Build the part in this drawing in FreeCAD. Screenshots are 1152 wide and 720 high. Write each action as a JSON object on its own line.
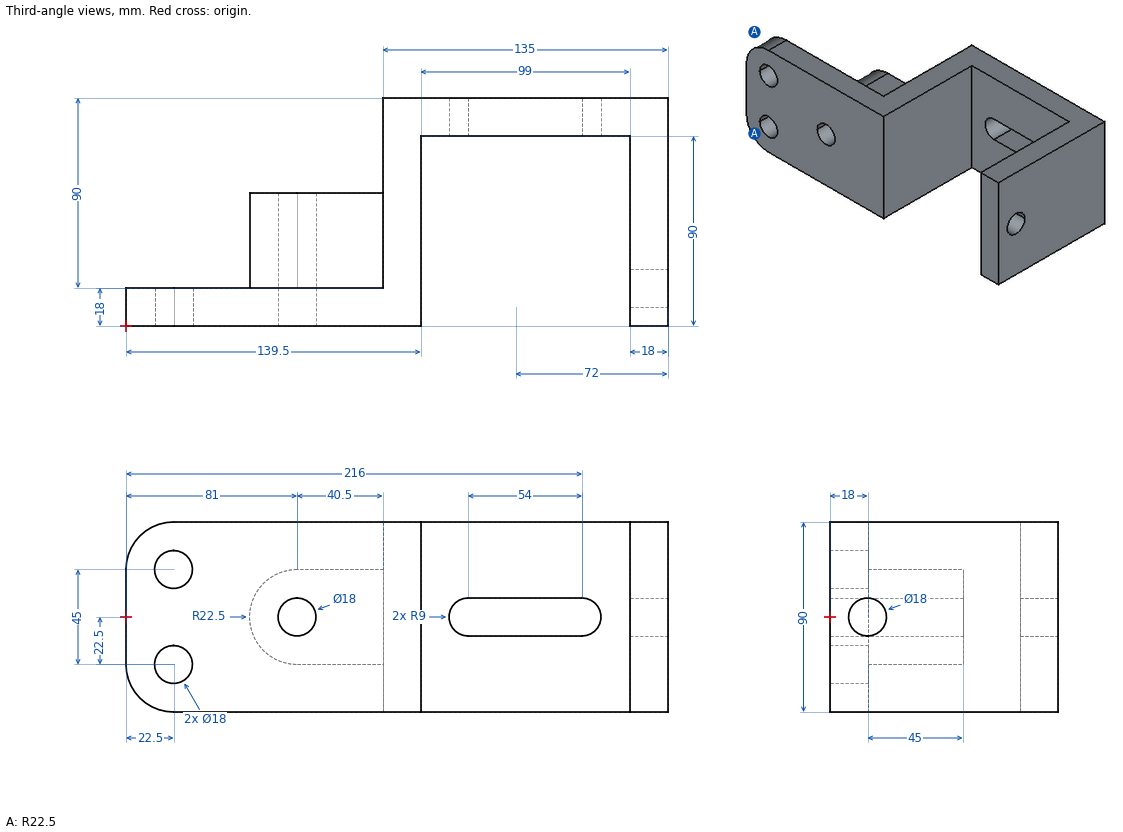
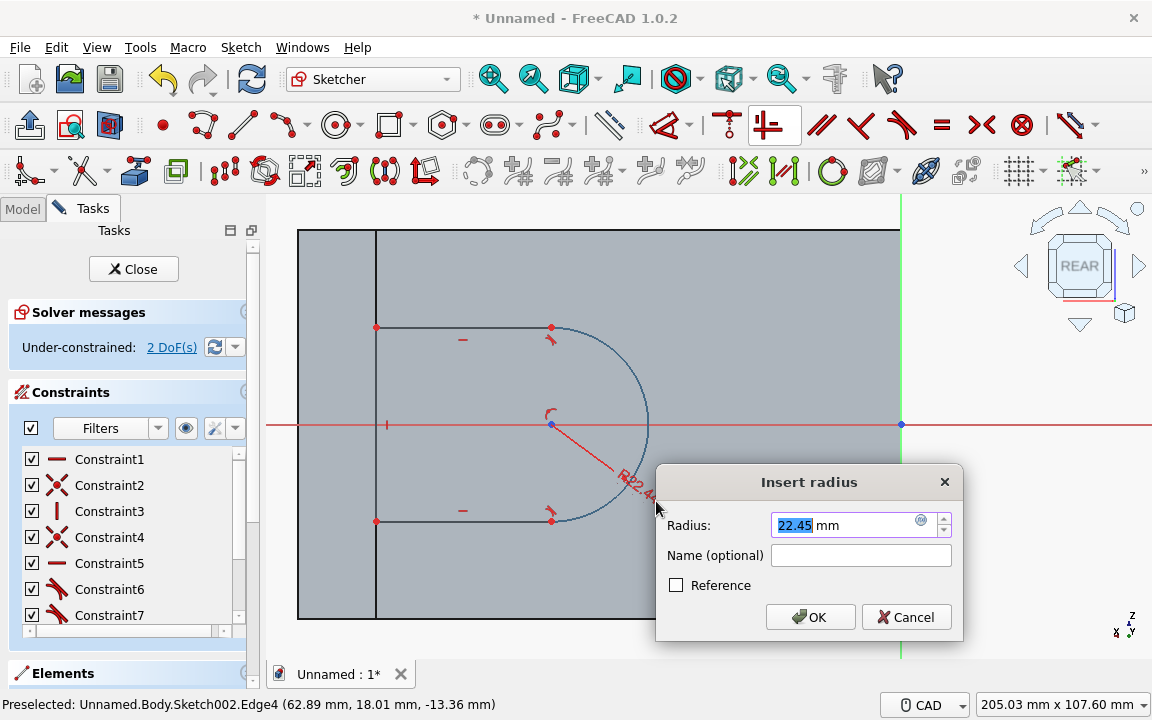
{"action": "type", "text": "22.5"}
{"action": "key", "text": "Return"}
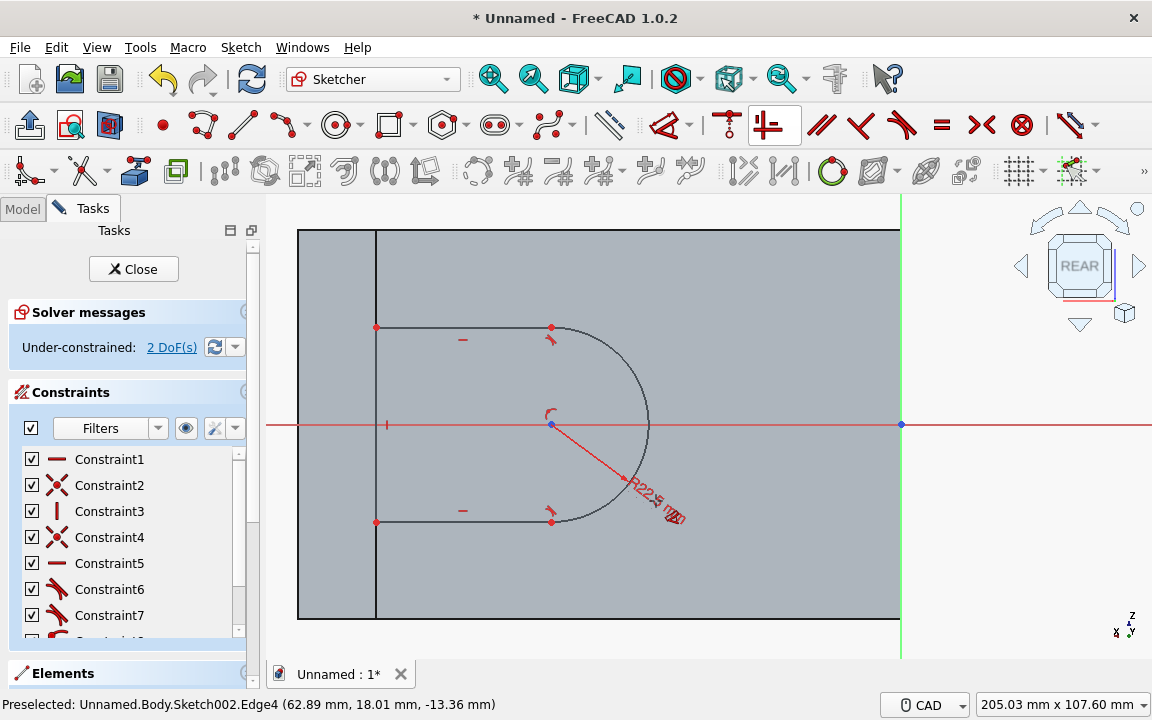
{"action": "left_click", "coordinate": [551, 328]}
{"action": "left_click", "coordinate": [726, 294]}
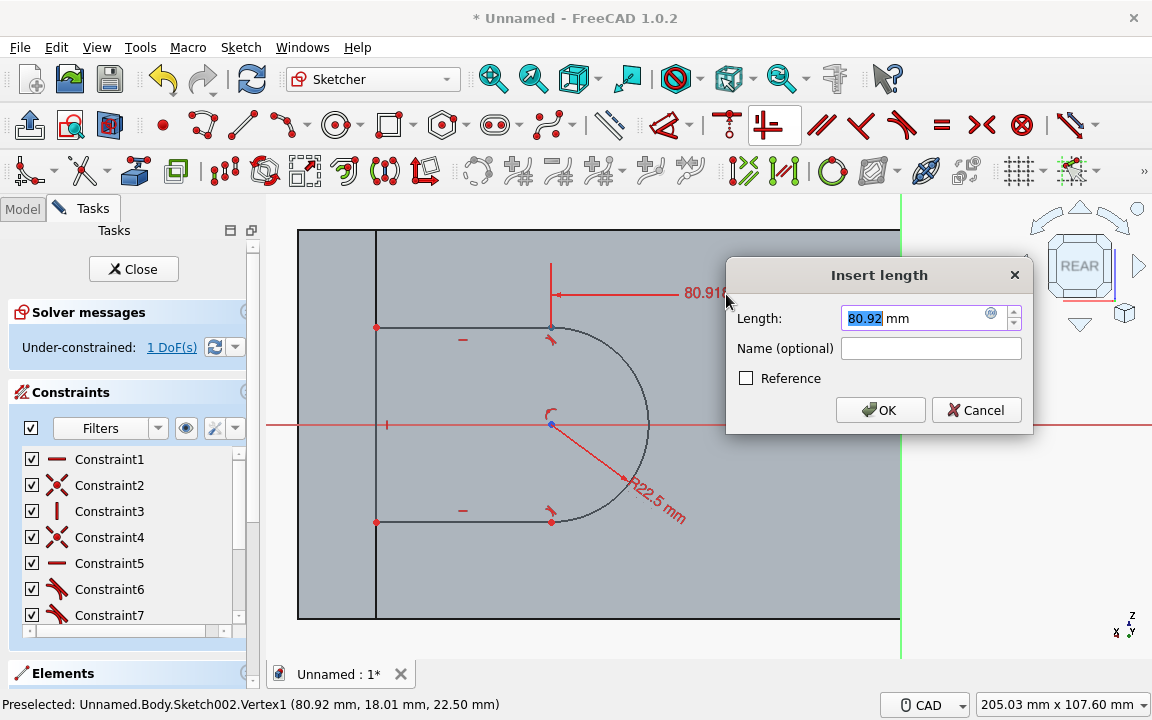
{"action": "type", "text": "81"}
{"action": "key", "text": "Return"}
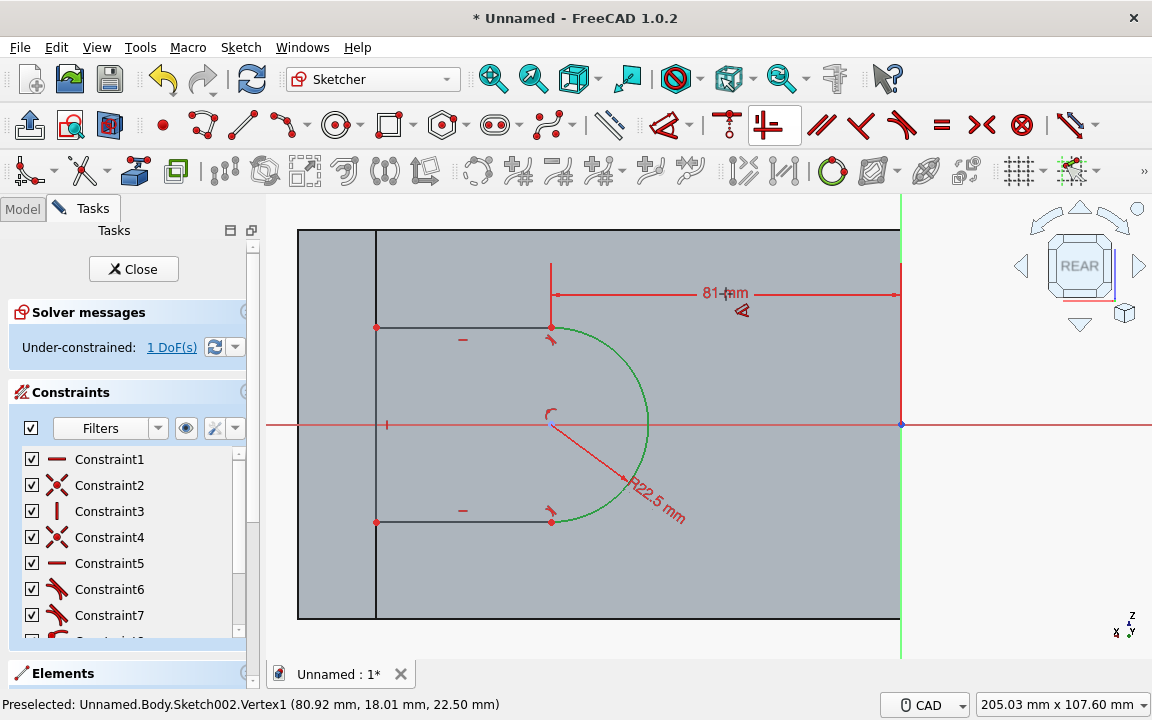
{"action": "left_click", "coordinate": [499, 328]}
{"action": "left_click", "coordinate": [464, 294]}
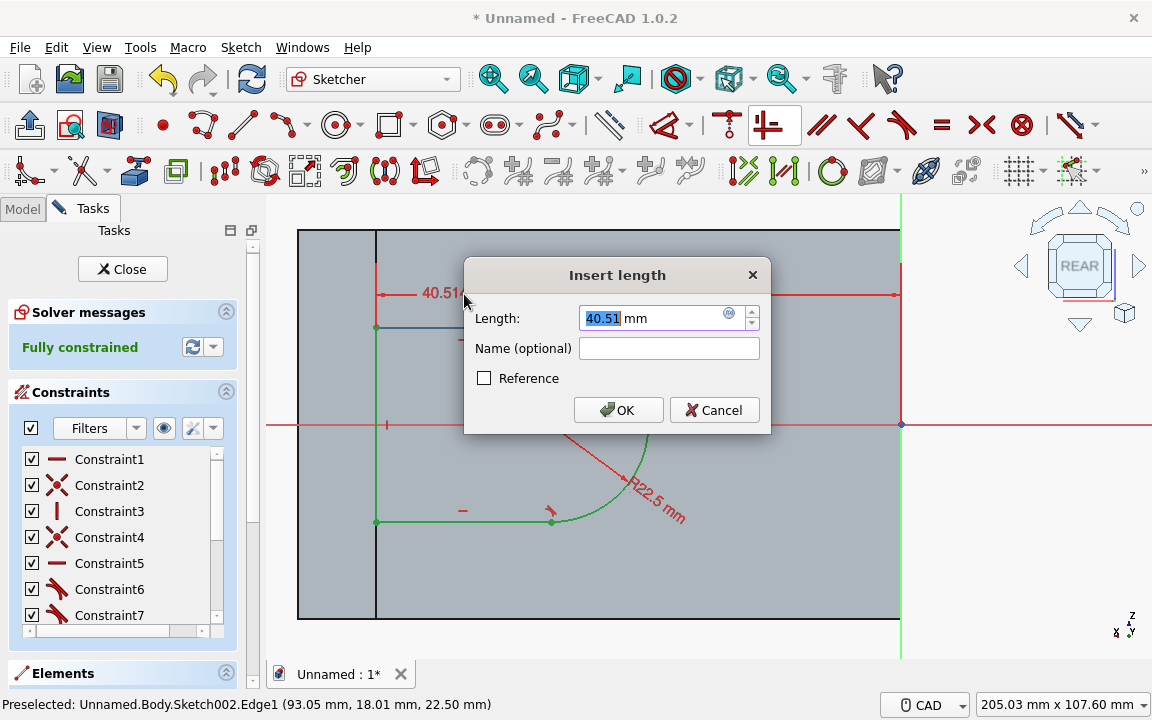
{"action": "type", "text": "40.5"}
{"action": "key", "text": "Return"}
{"action": "key", "text": "Escape"}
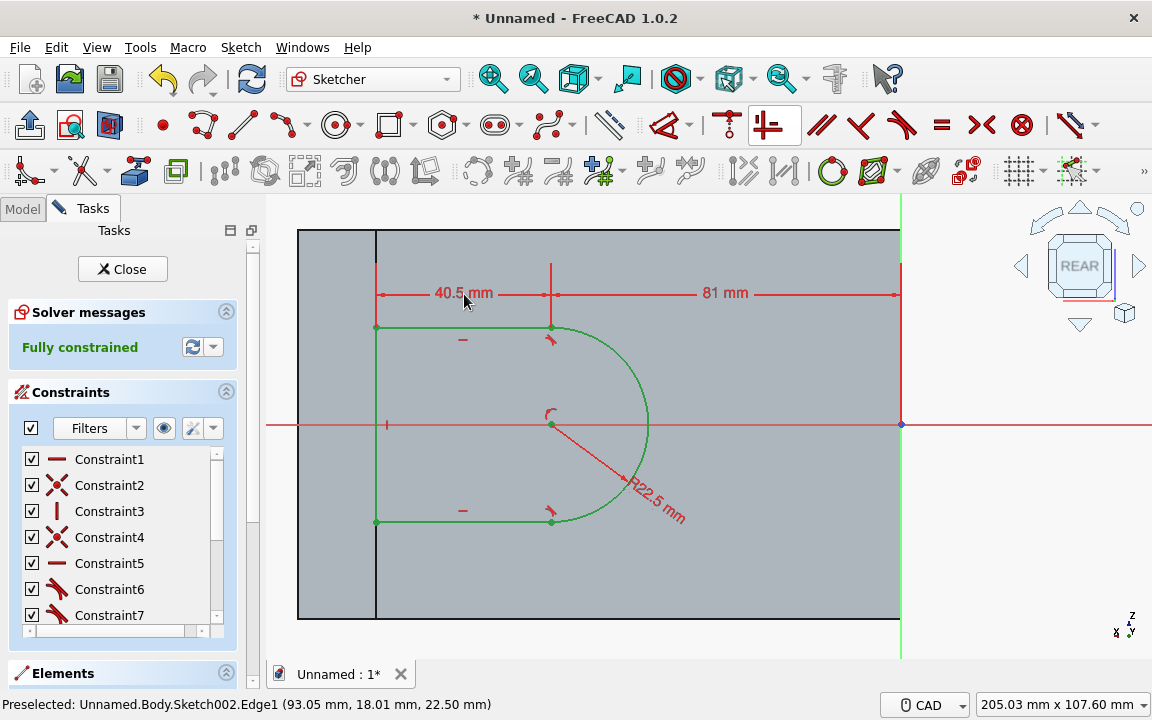
{"action": "left_click", "coordinate": [123, 269]}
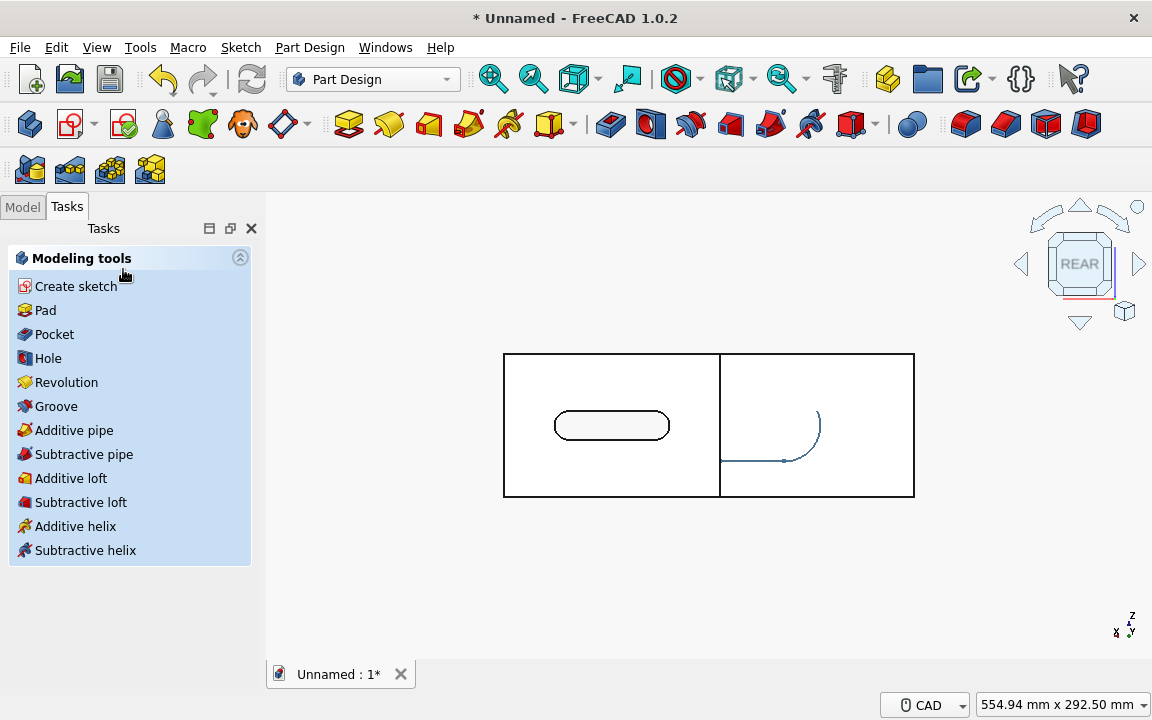
{"action": "left_click", "coordinate": [350, 124]}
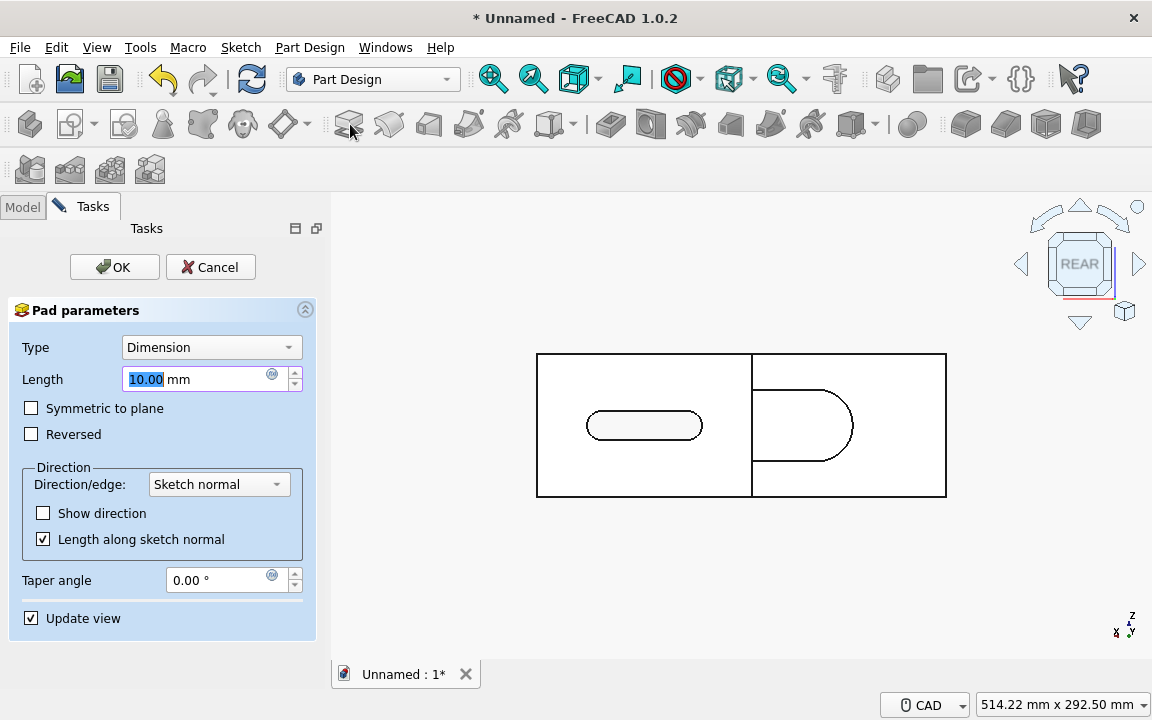
{"action": "type", "text": "45"}
{"action": "key", "text": "Tab"}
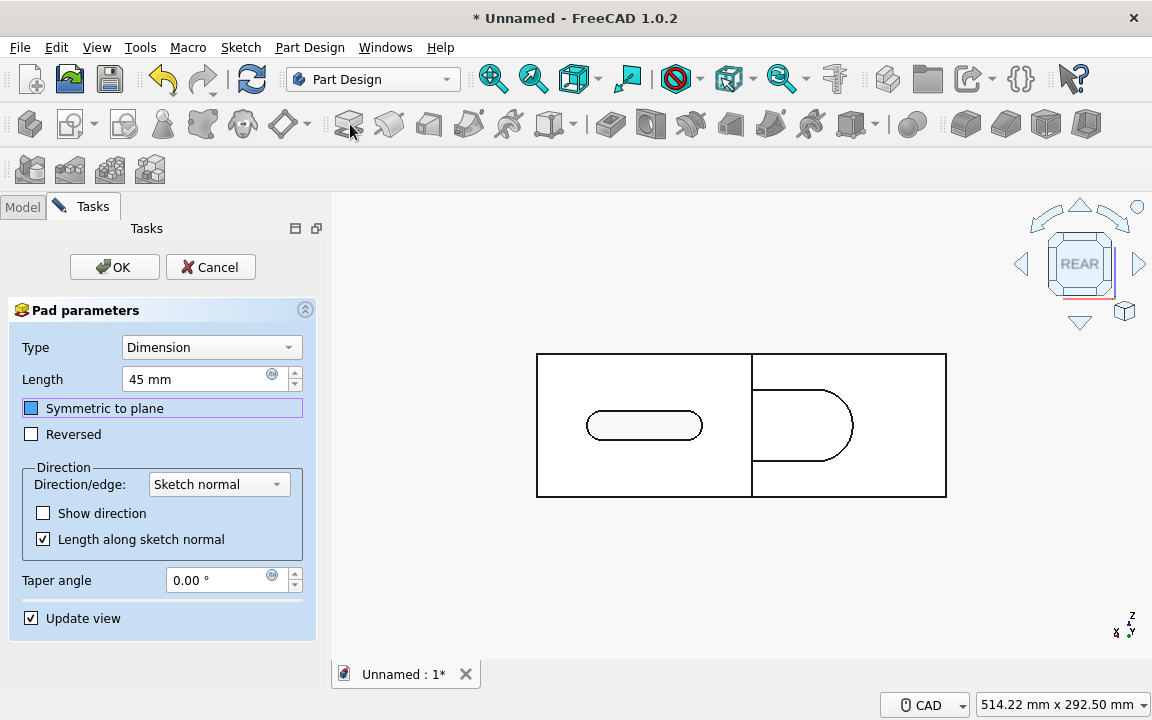
{"action": "left_click", "coordinate": [115, 267]}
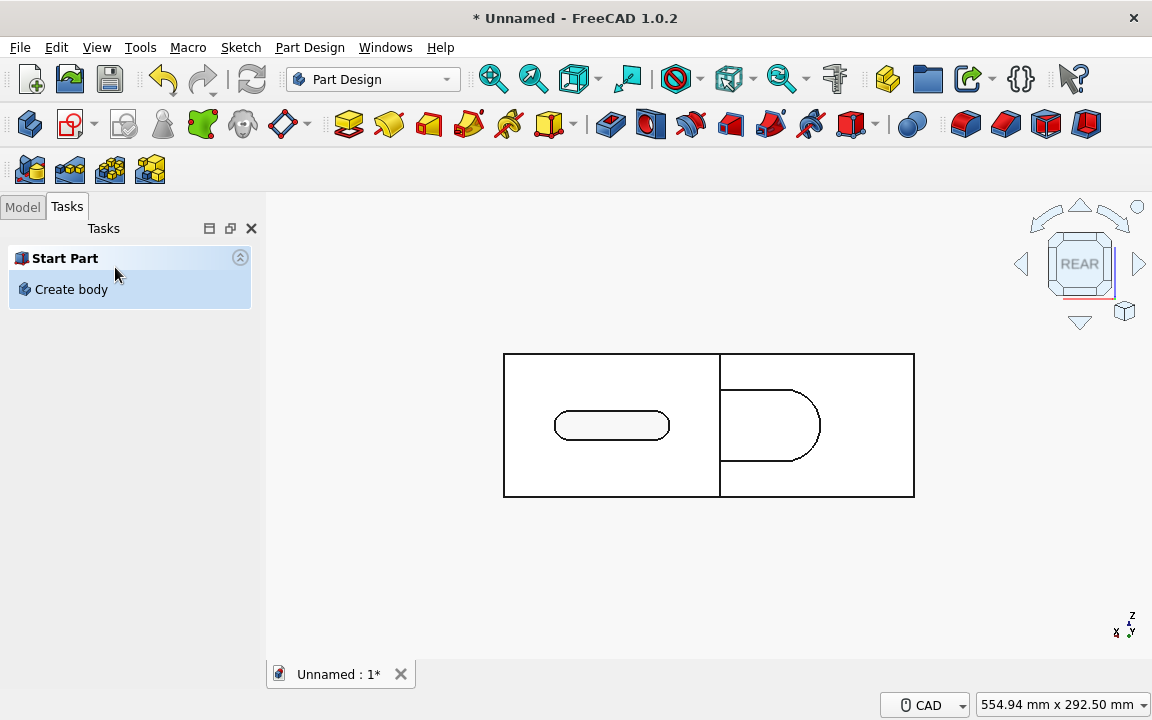
{"action": "left_click", "coordinate": [756, 424]}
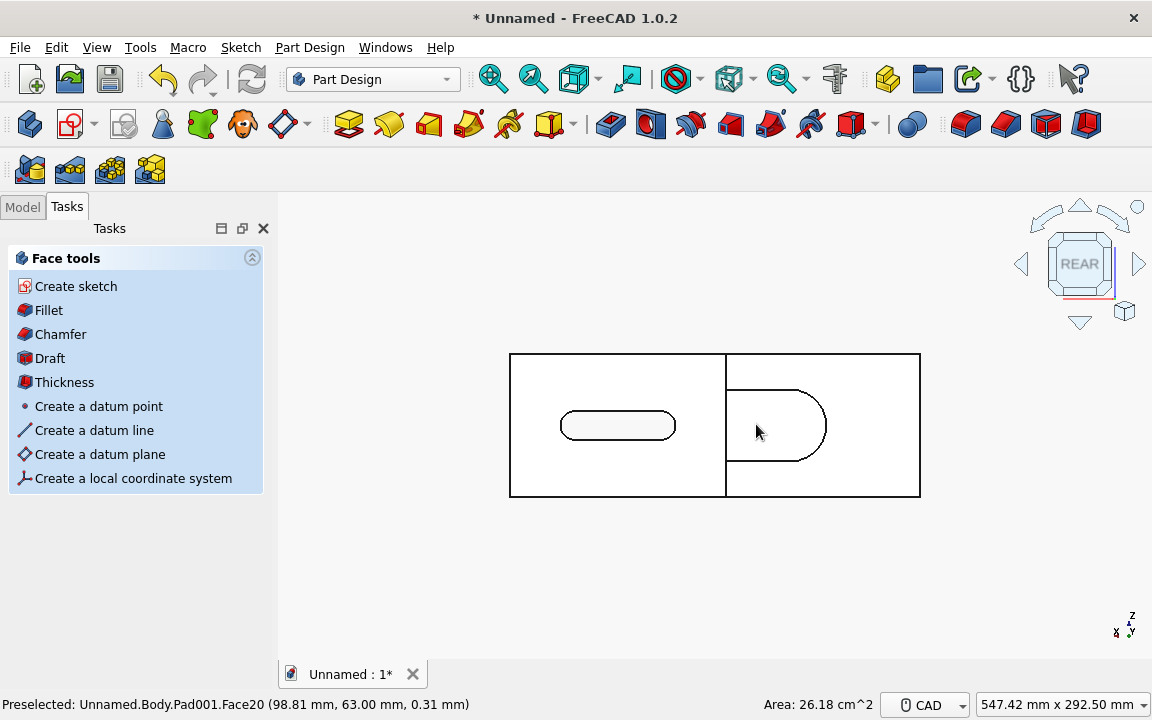
{"action": "left_click", "coordinate": [70, 124]}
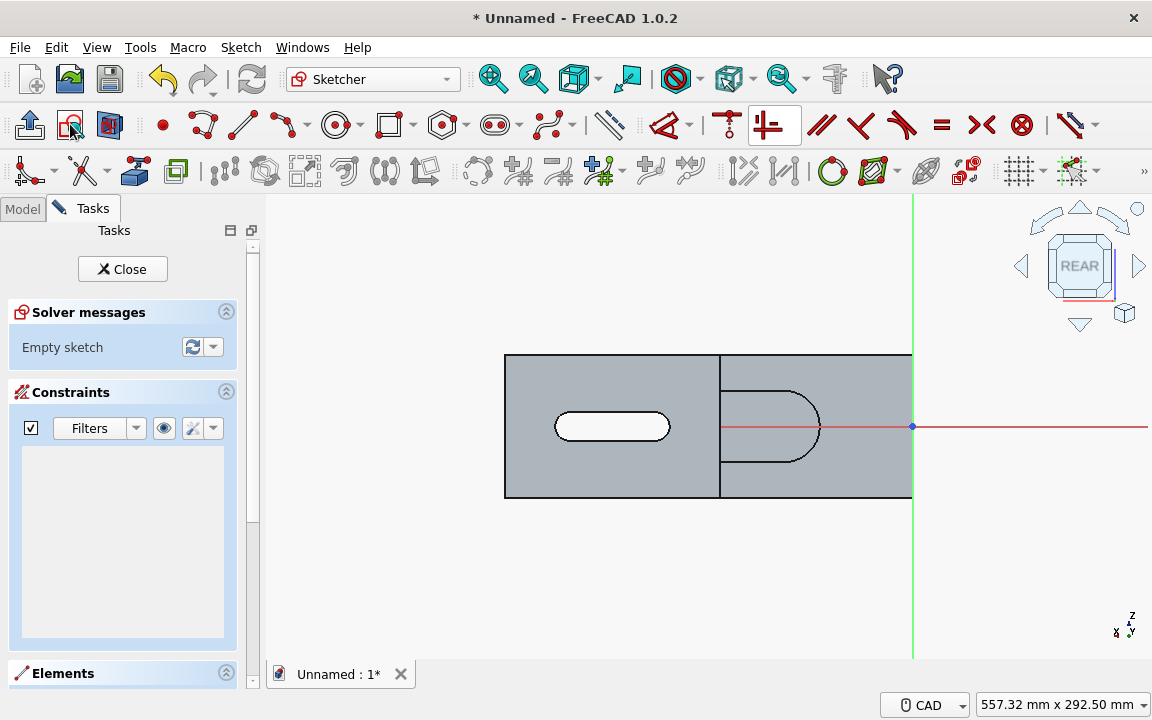
{"action": "scroll", "coordinate": [798, 427], "scroll_direction": "up", "scroll_amount": 12}